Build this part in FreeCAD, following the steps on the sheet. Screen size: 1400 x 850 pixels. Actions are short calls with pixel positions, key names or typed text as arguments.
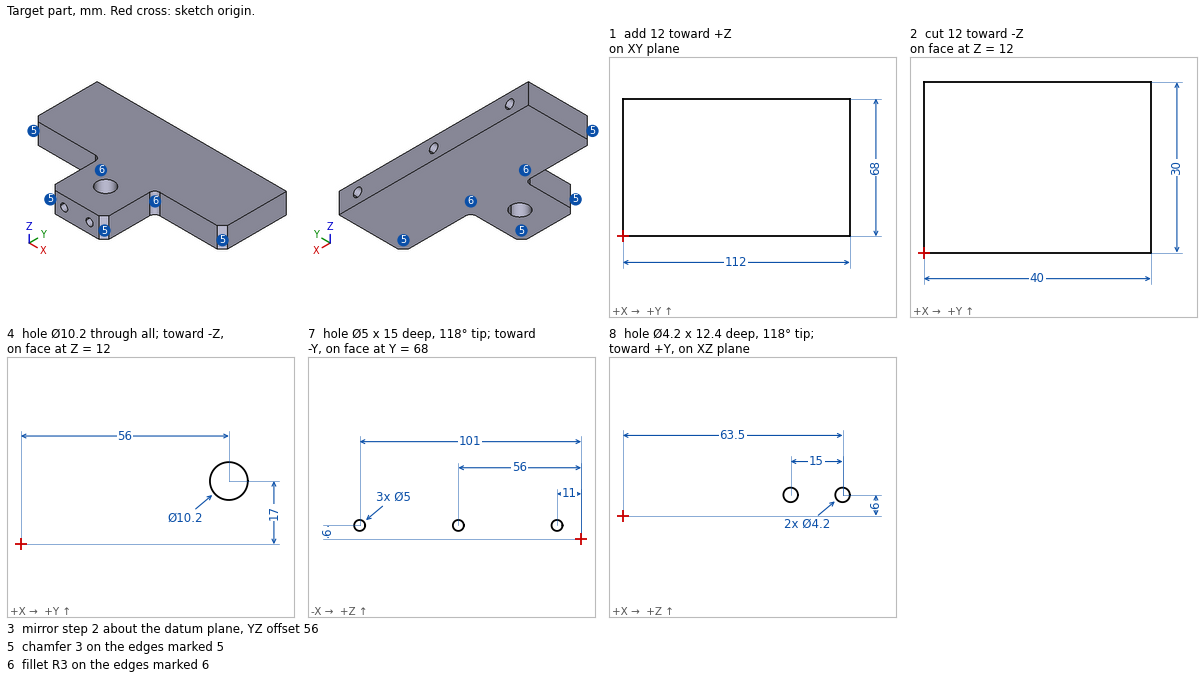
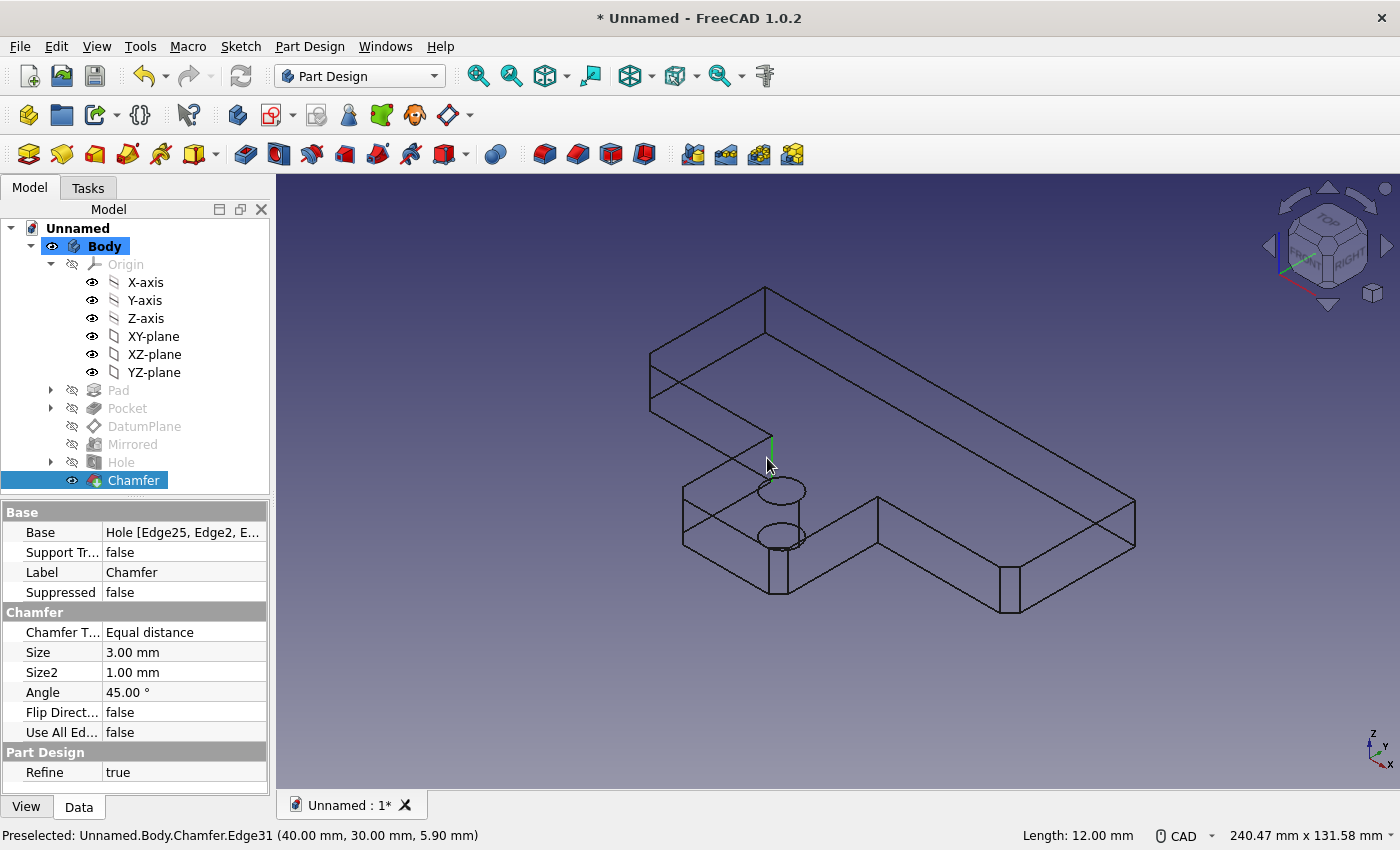
click(878, 519, ctrl)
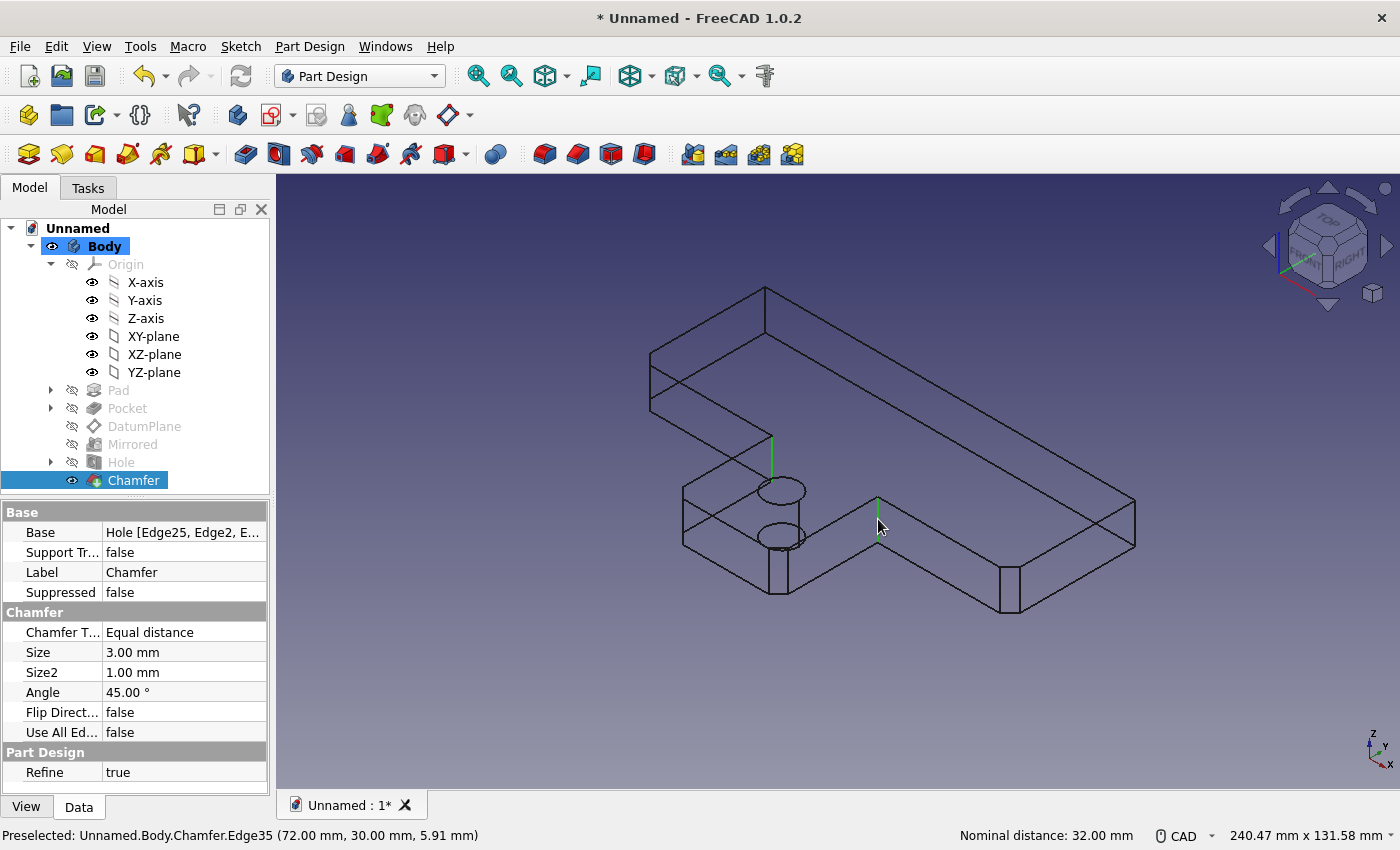
key(v)
key(1)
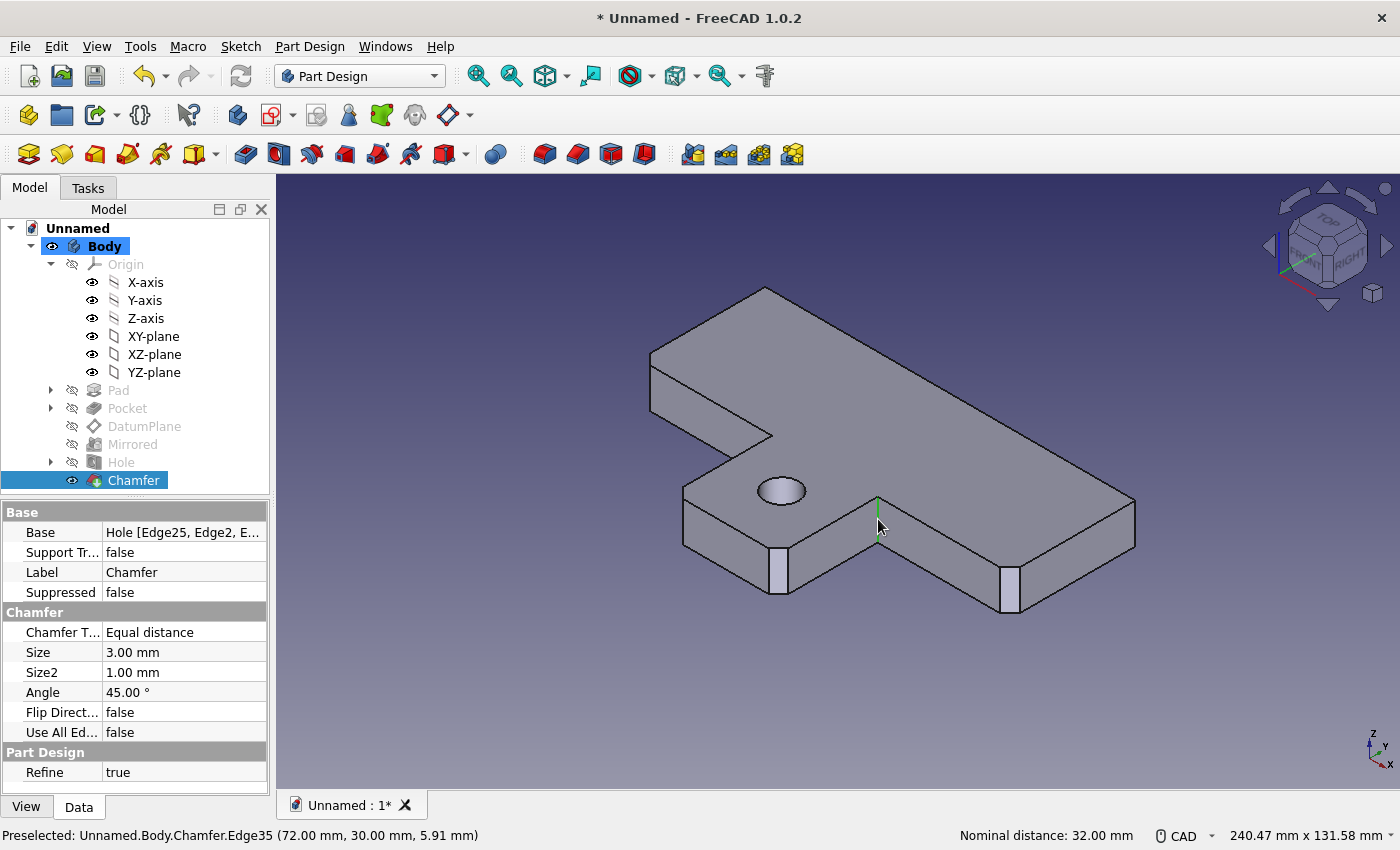
click(545, 154)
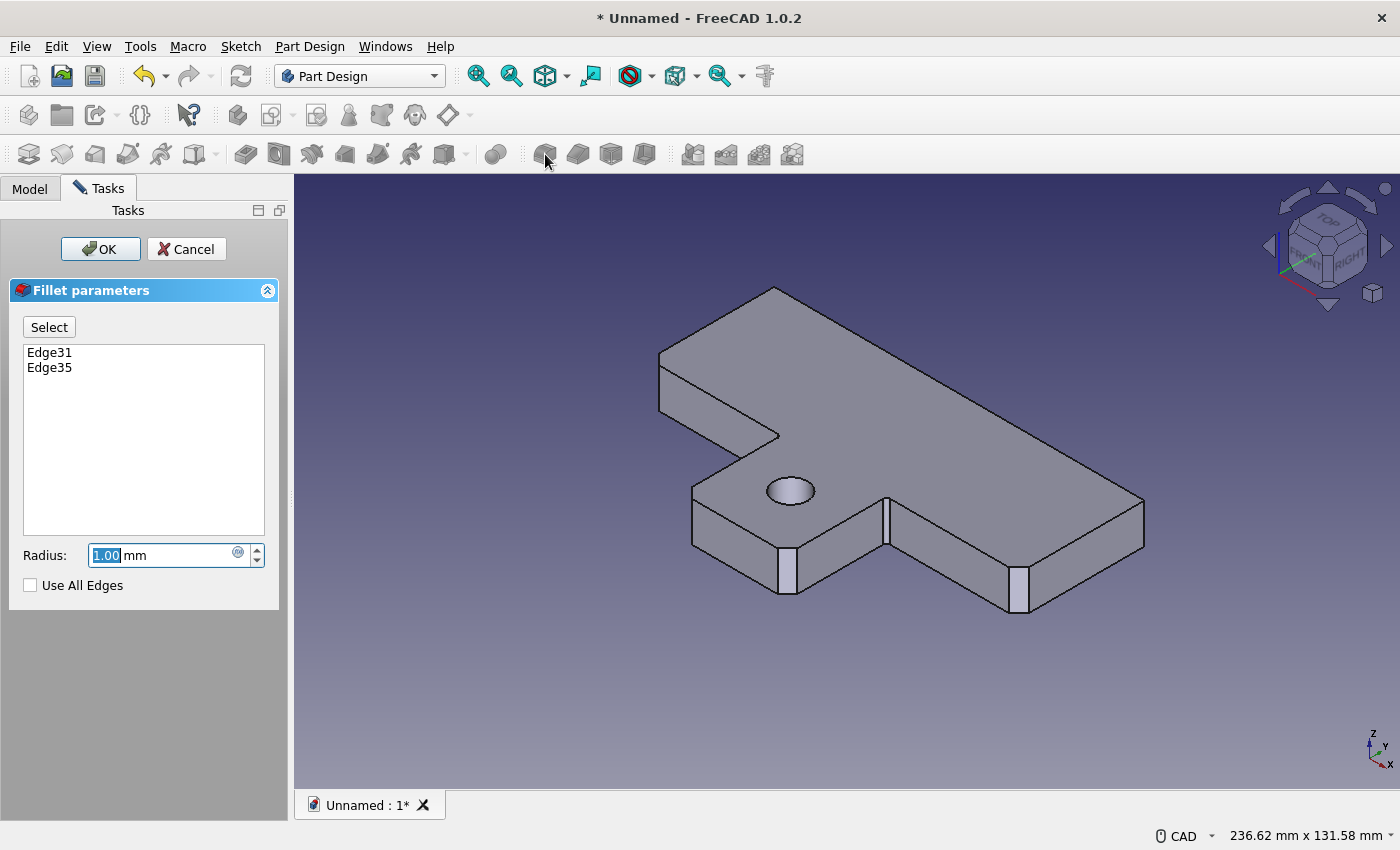
text(3)
key(Tab)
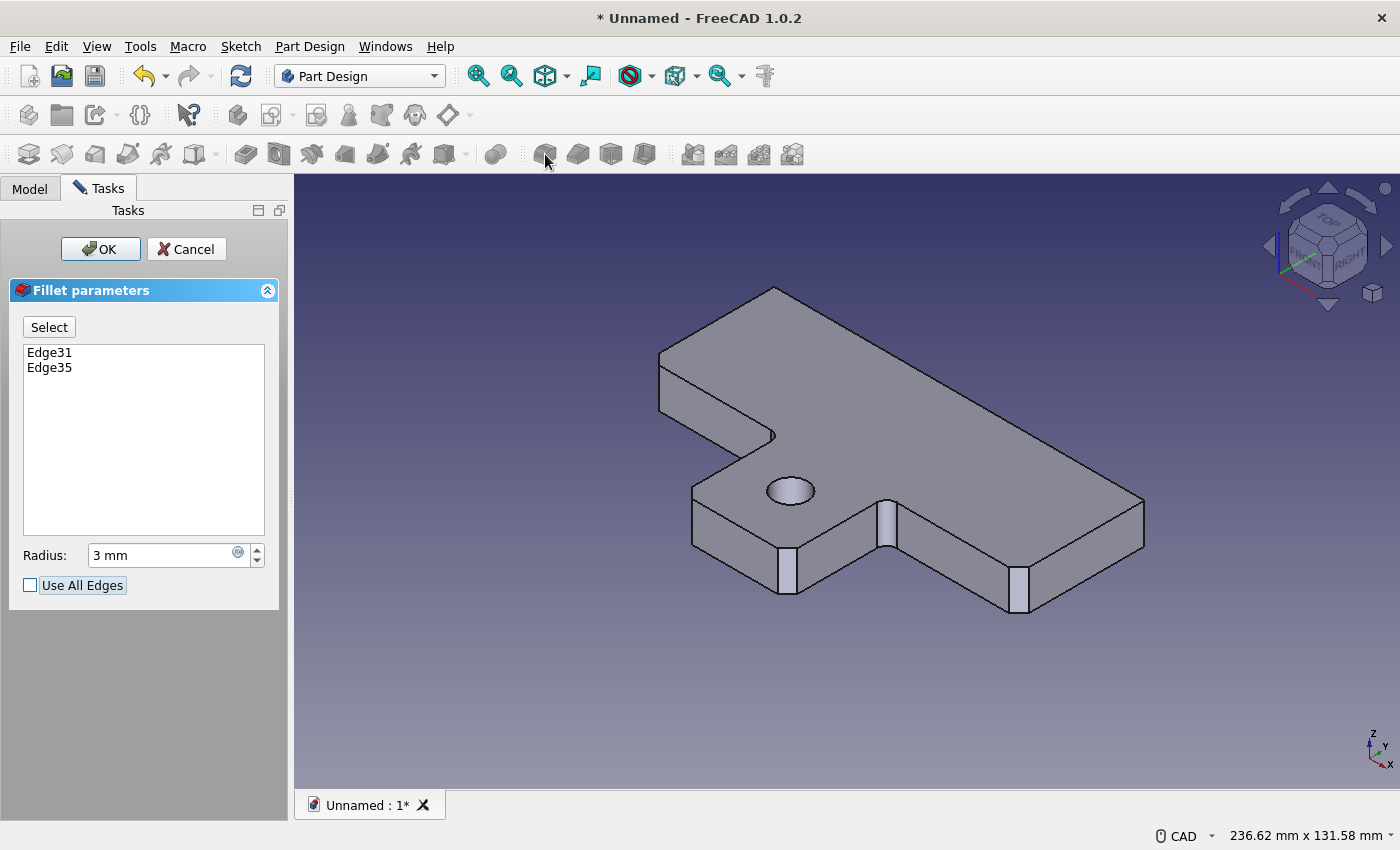
click(101, 249)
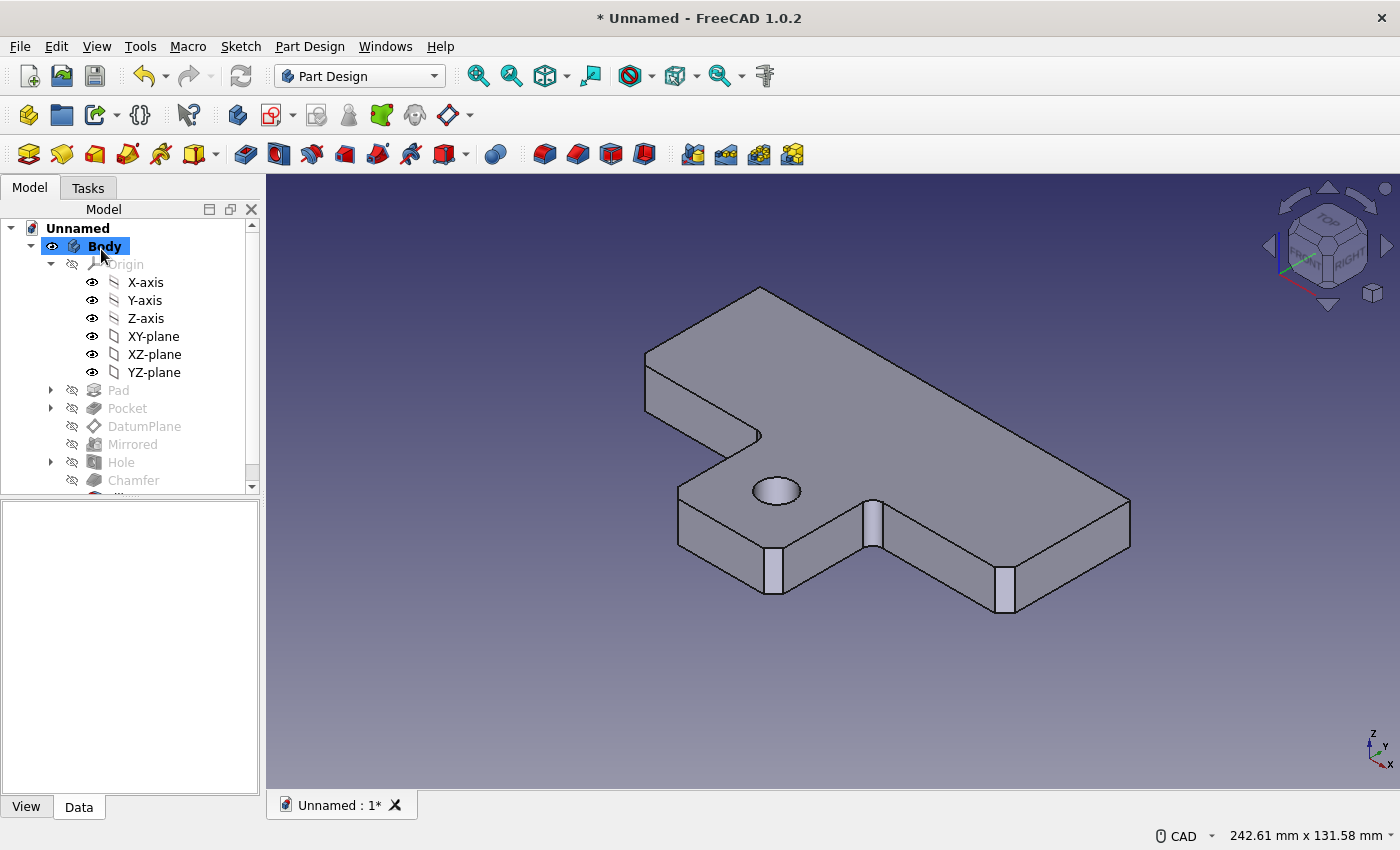
key(4)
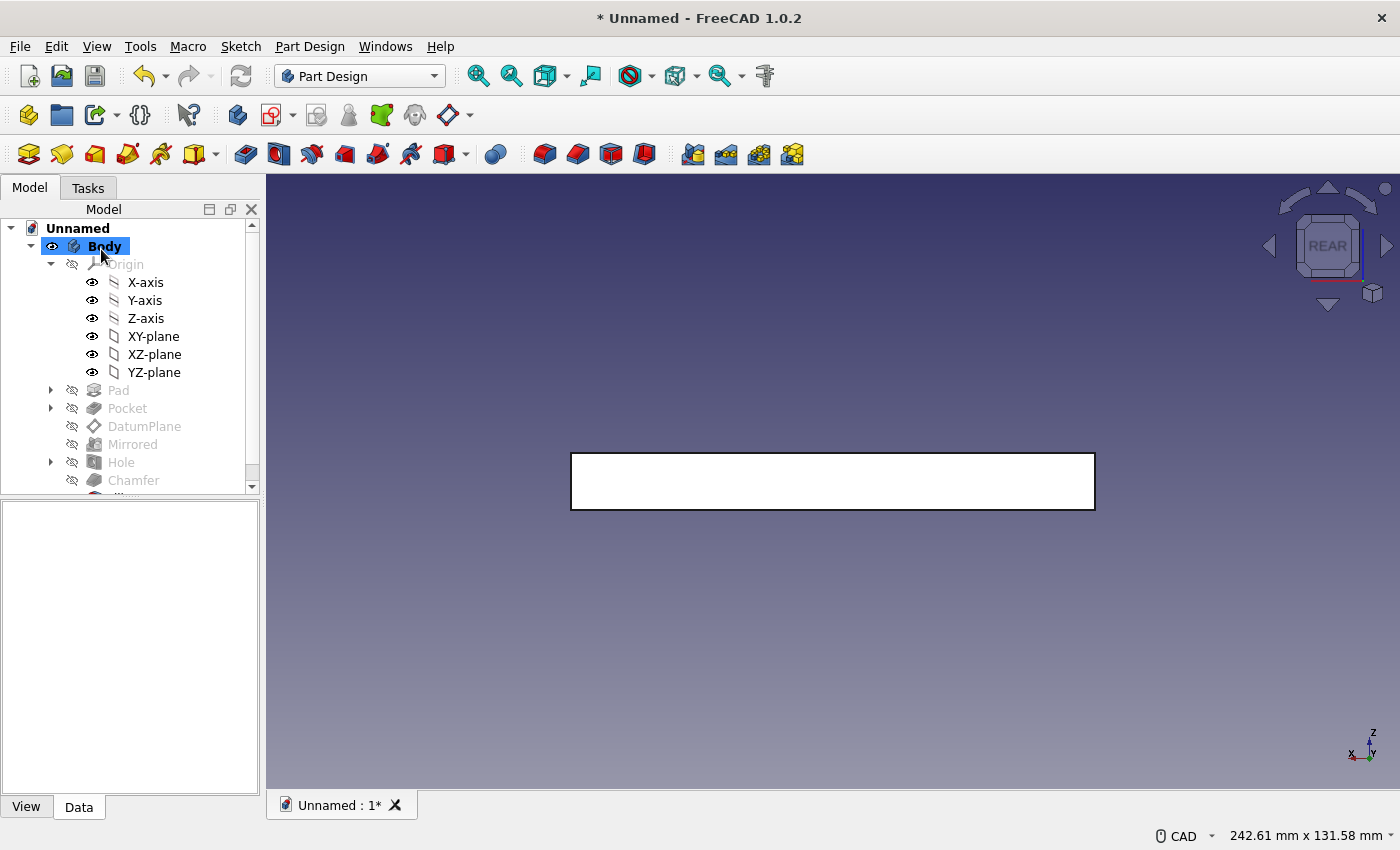
click(609, 480)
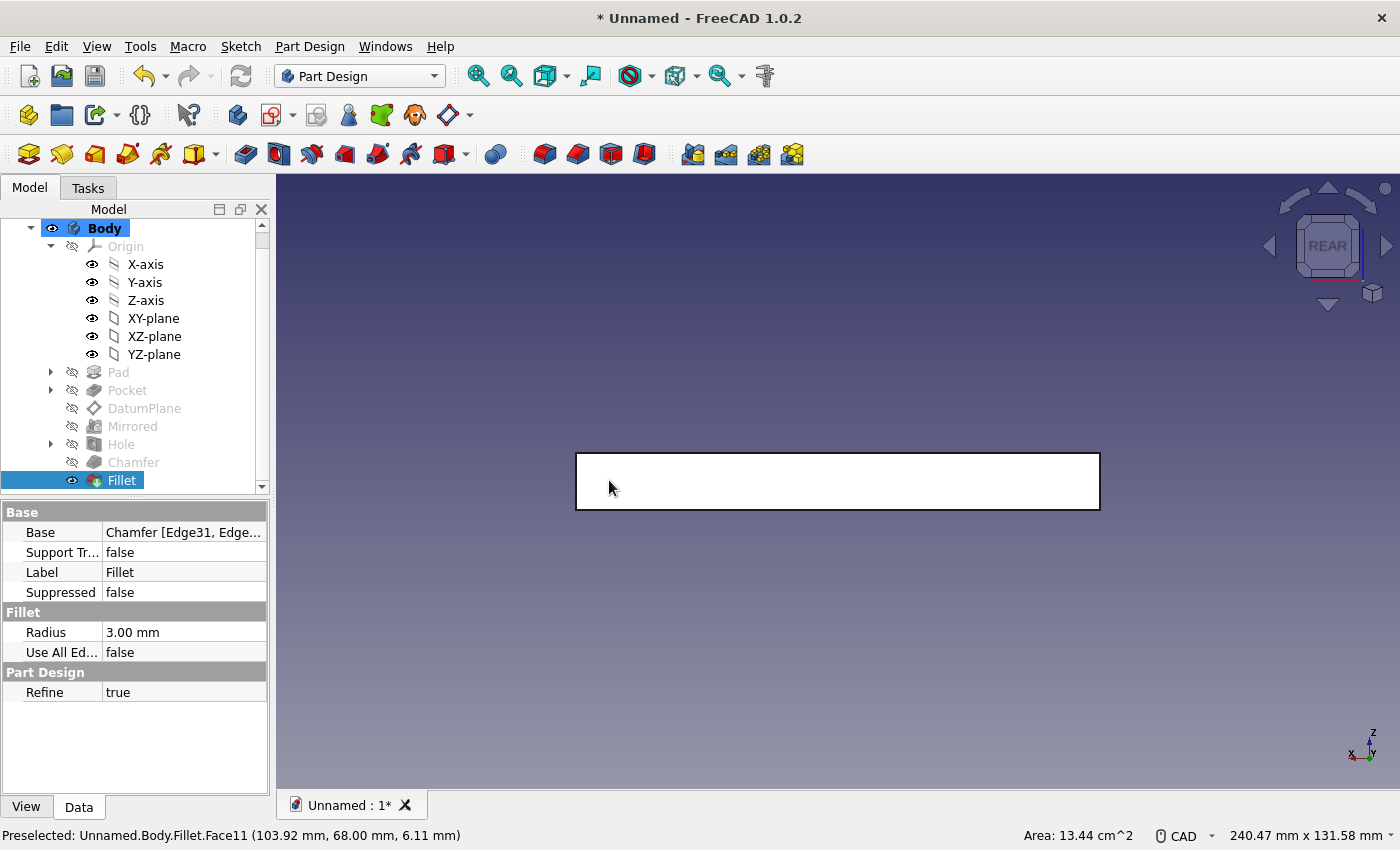
click(270, 116)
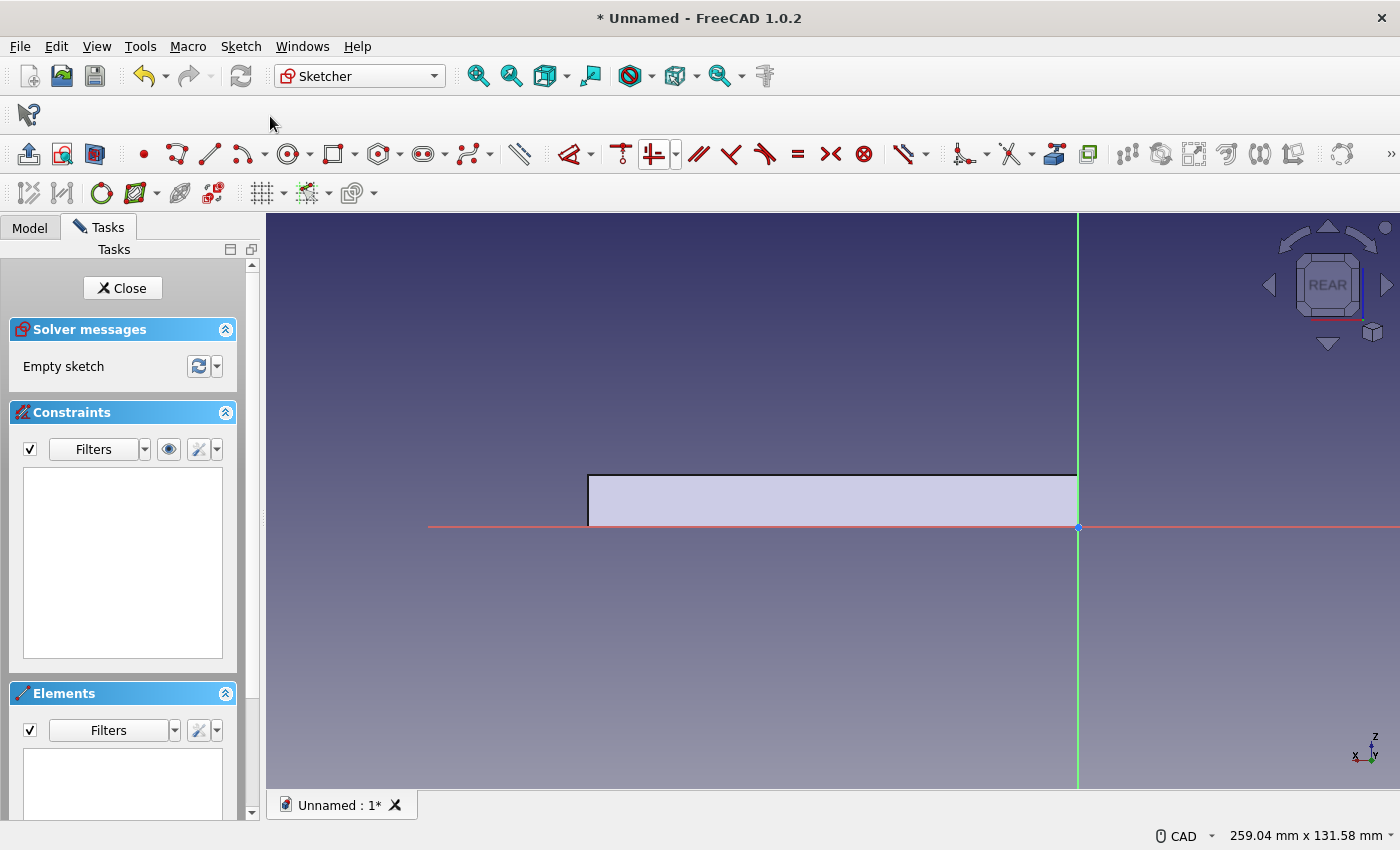
scroll(1029, 524, up, 2)